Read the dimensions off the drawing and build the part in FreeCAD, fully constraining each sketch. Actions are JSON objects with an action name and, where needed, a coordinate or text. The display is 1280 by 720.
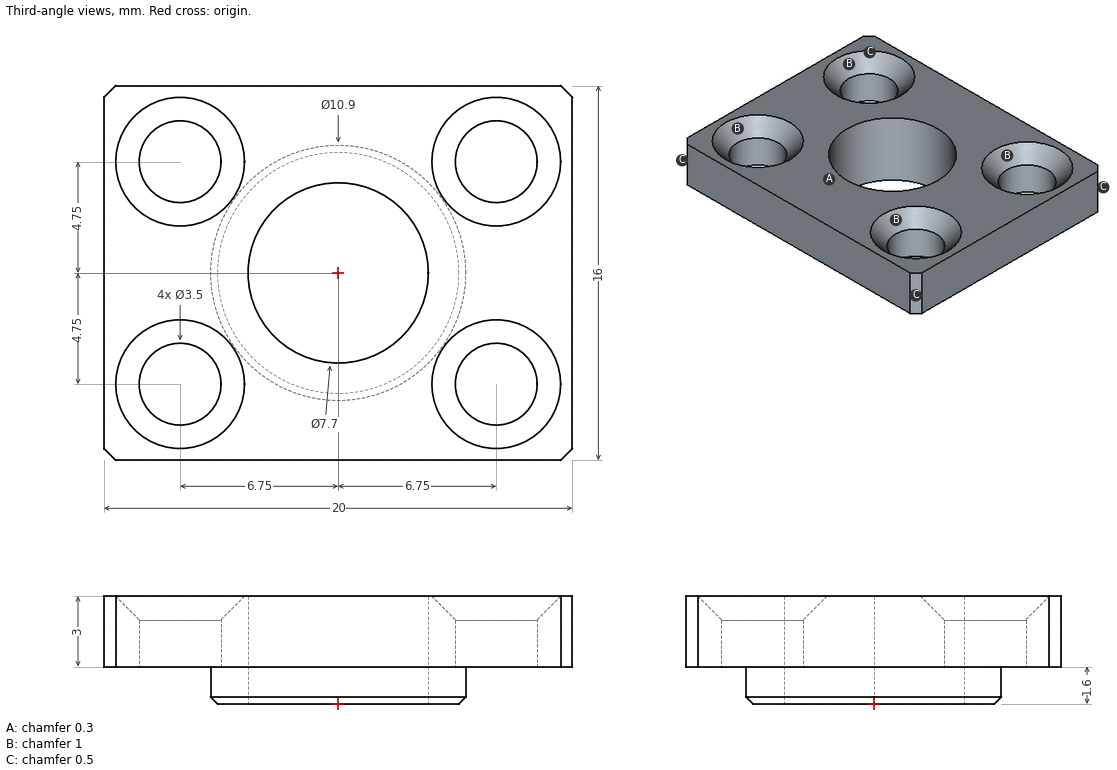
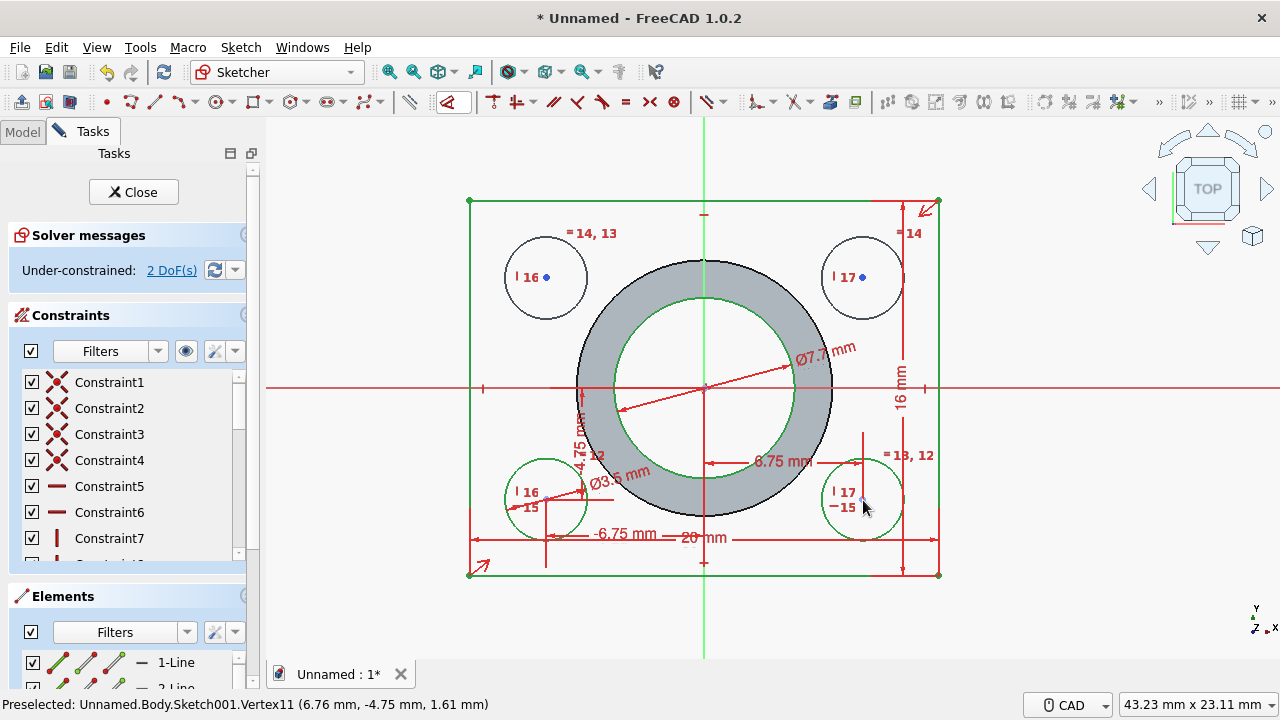
{"action": "left_click", "coordinate": [546, 278]}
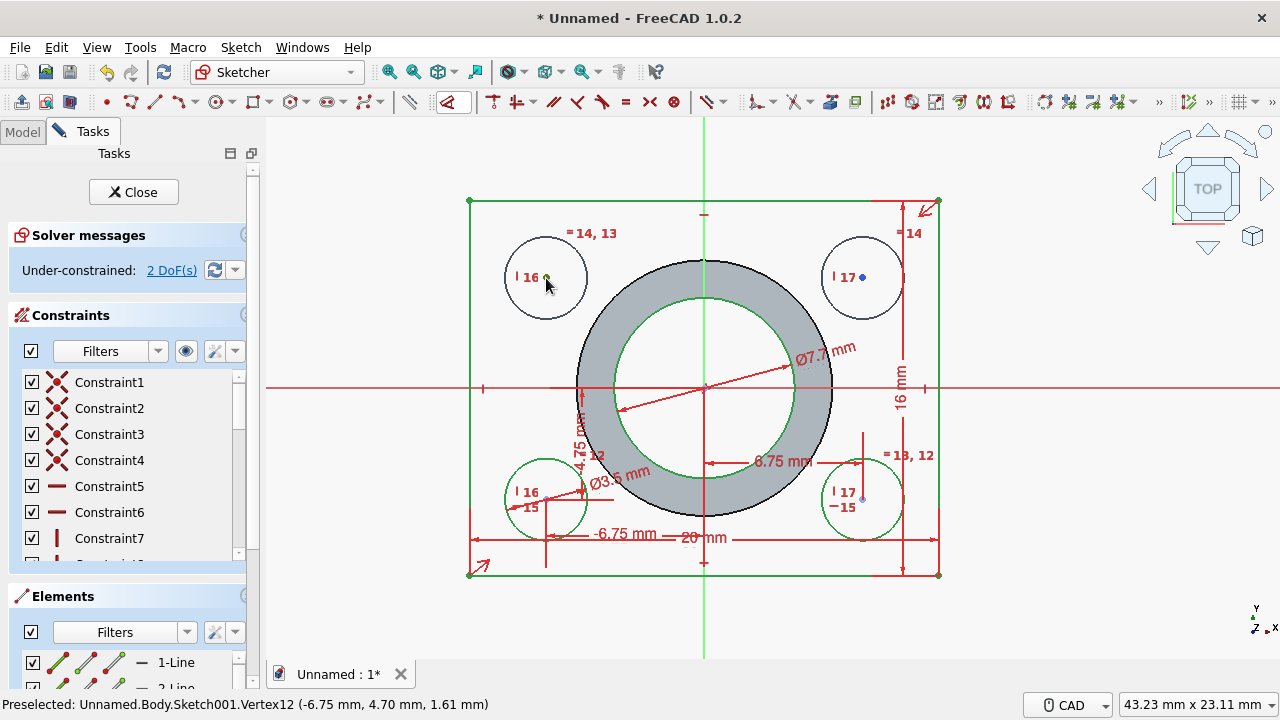
{"action": "key", "text": "i"}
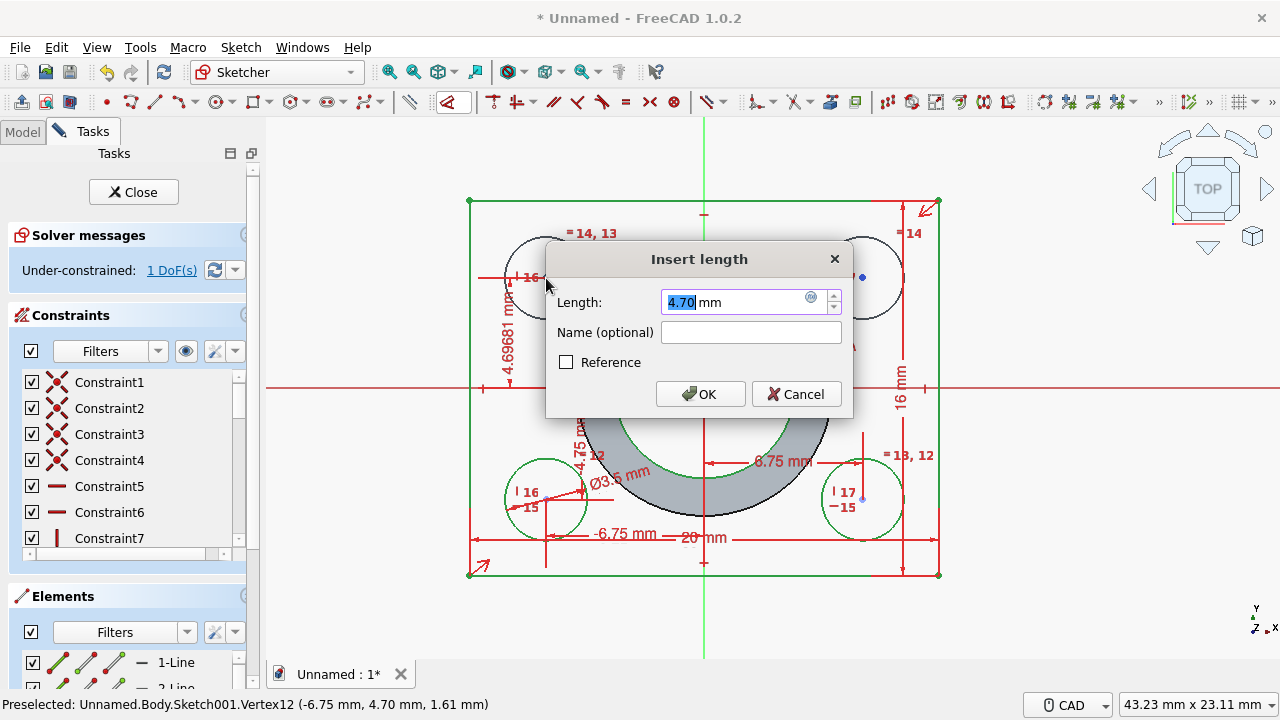
{"action": "type", "text": "4.75"}
{"action": "key", "text": "Return"}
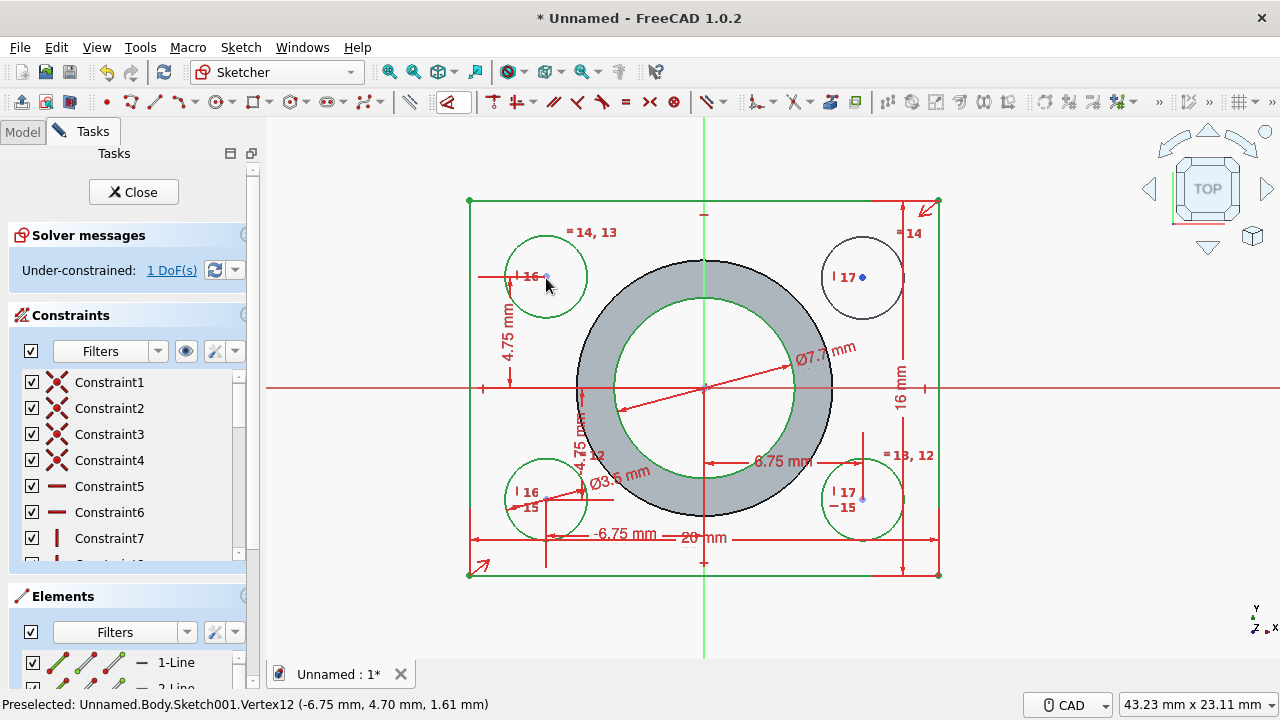
{"action": "left_click", "coordinate": [863, 278]}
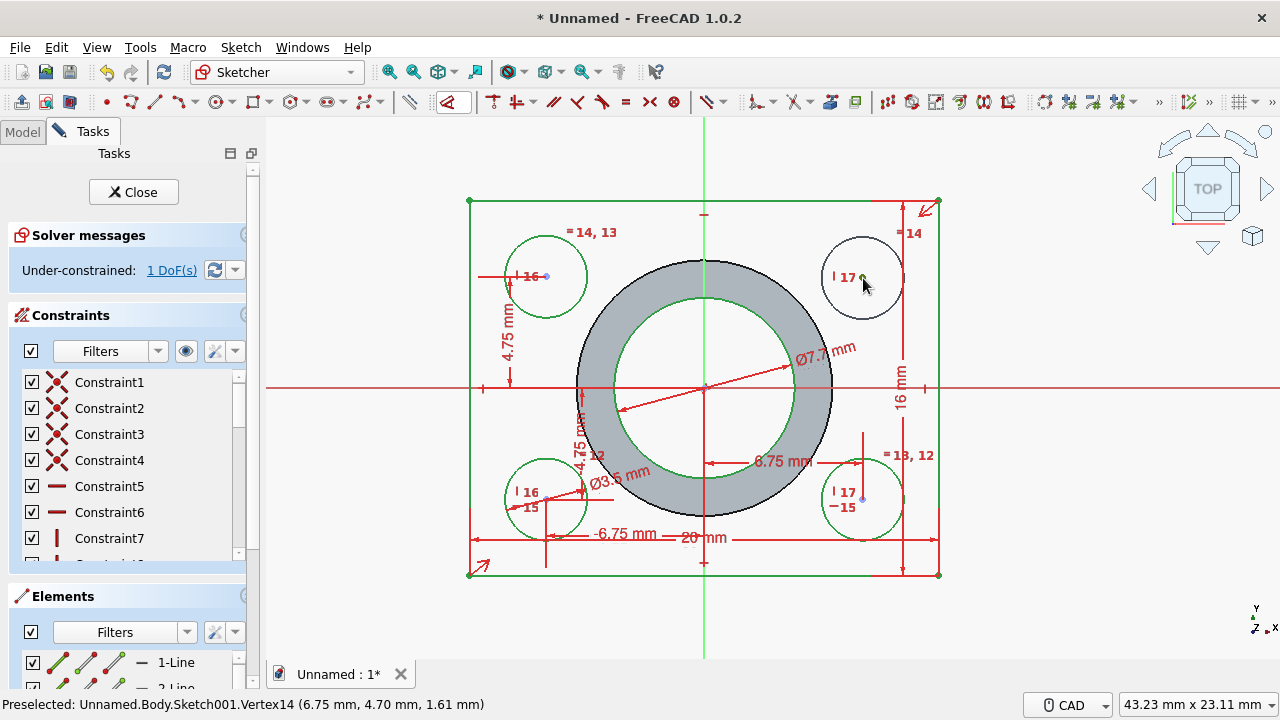
{"action": "key", "text": "i"}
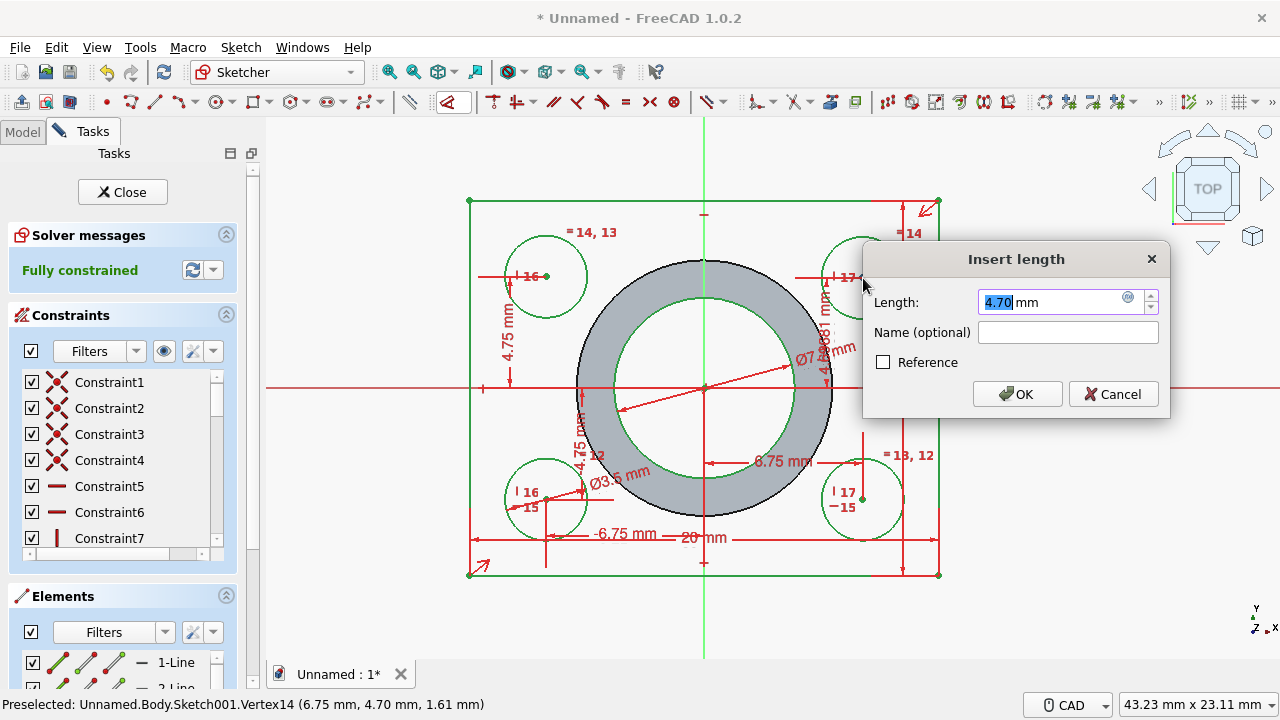
{"action": "type", "text": "4.75"}
{"action": "key", "text": "Return"}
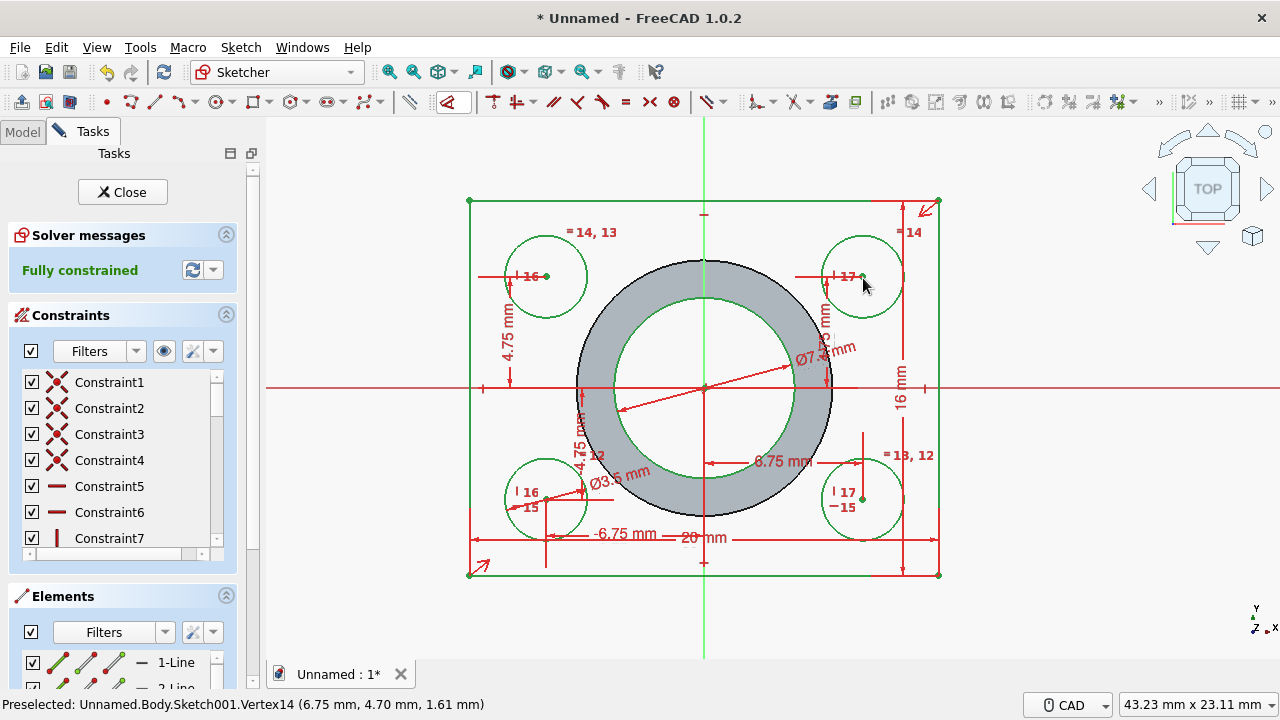
{"action": "left_click", "coordinate": [123, 192]}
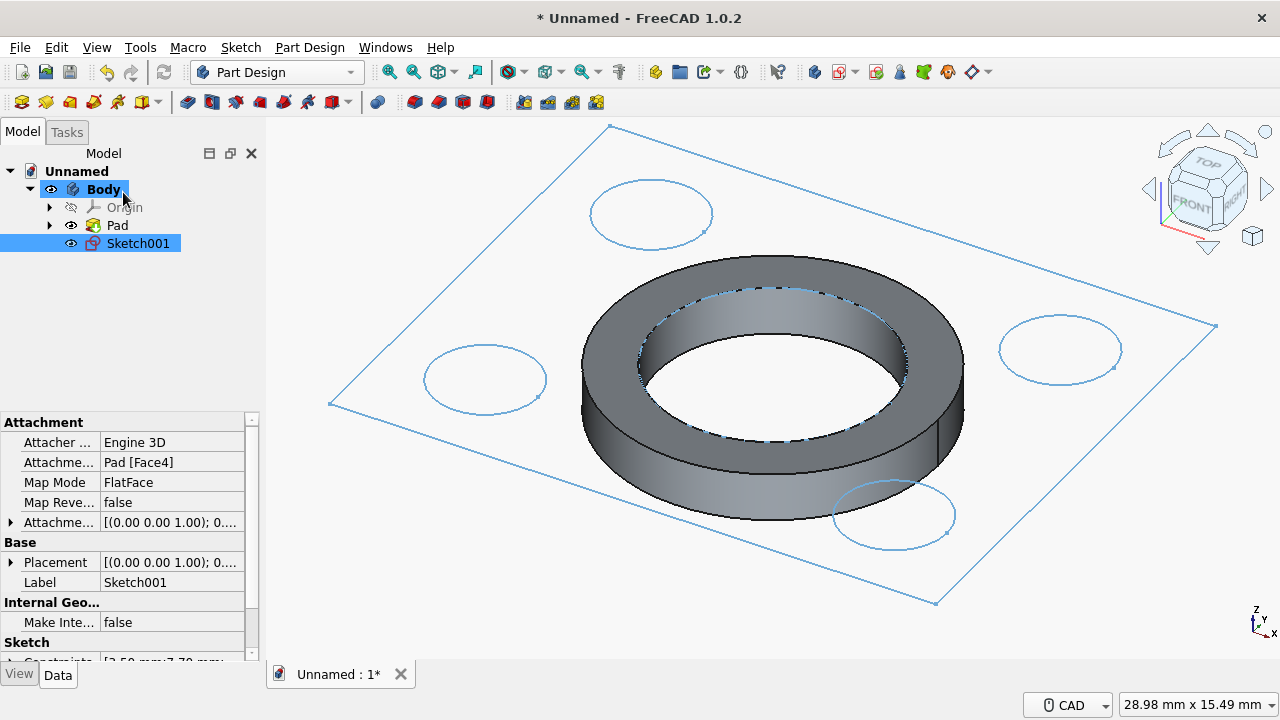
{"action": "left_click", "coordinate": [22, 102]}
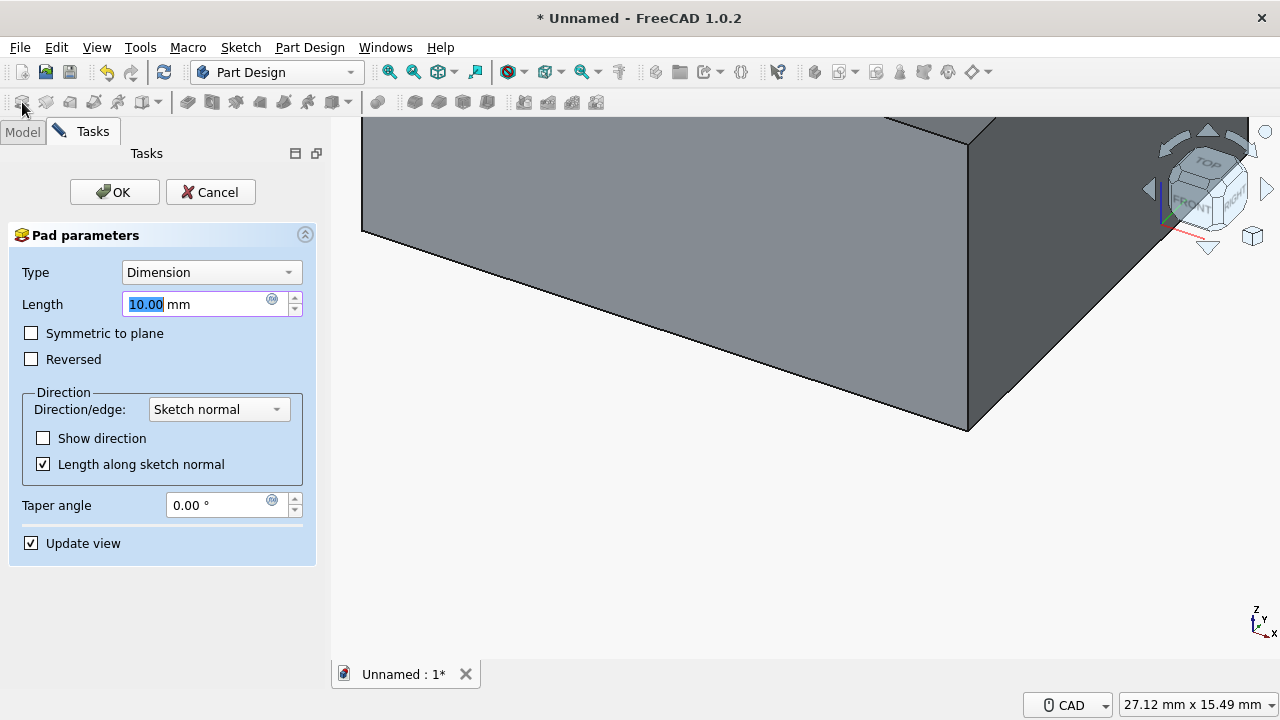
{"action": "type", "text": "3"}
{"action": "key", "text": "Tab"}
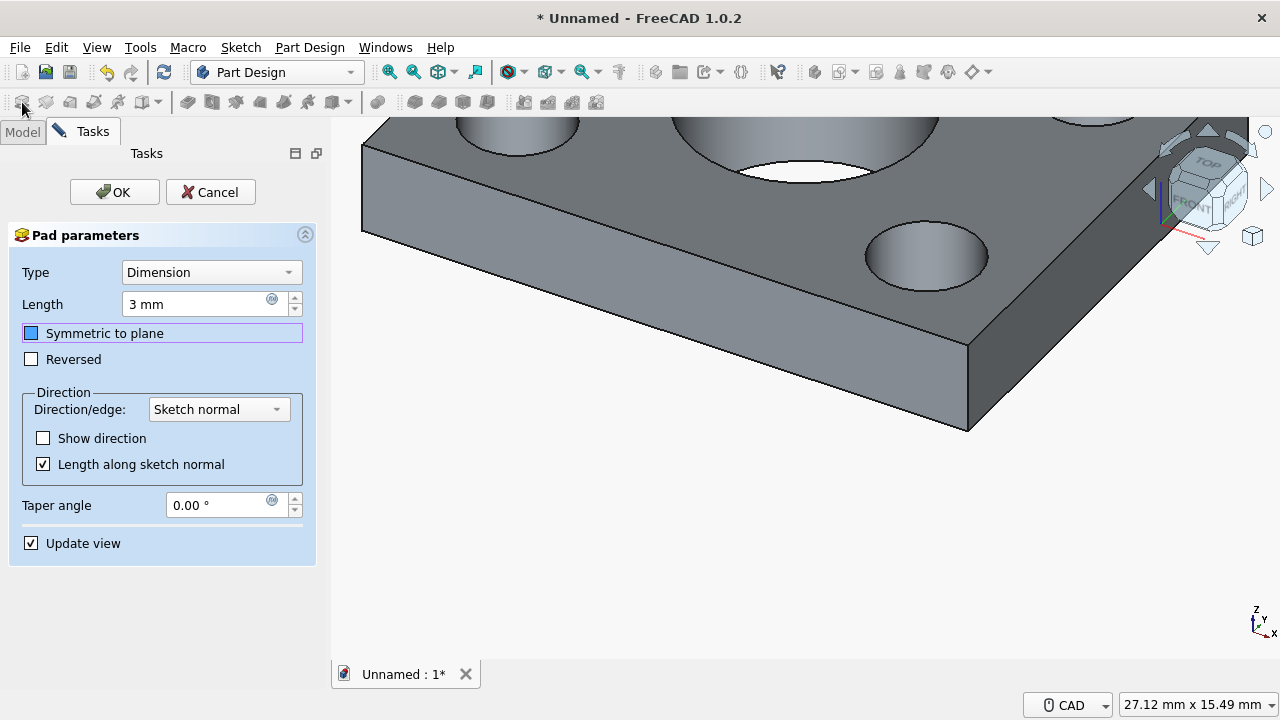
{"action": "left_click", "coordinate": [115, 192]}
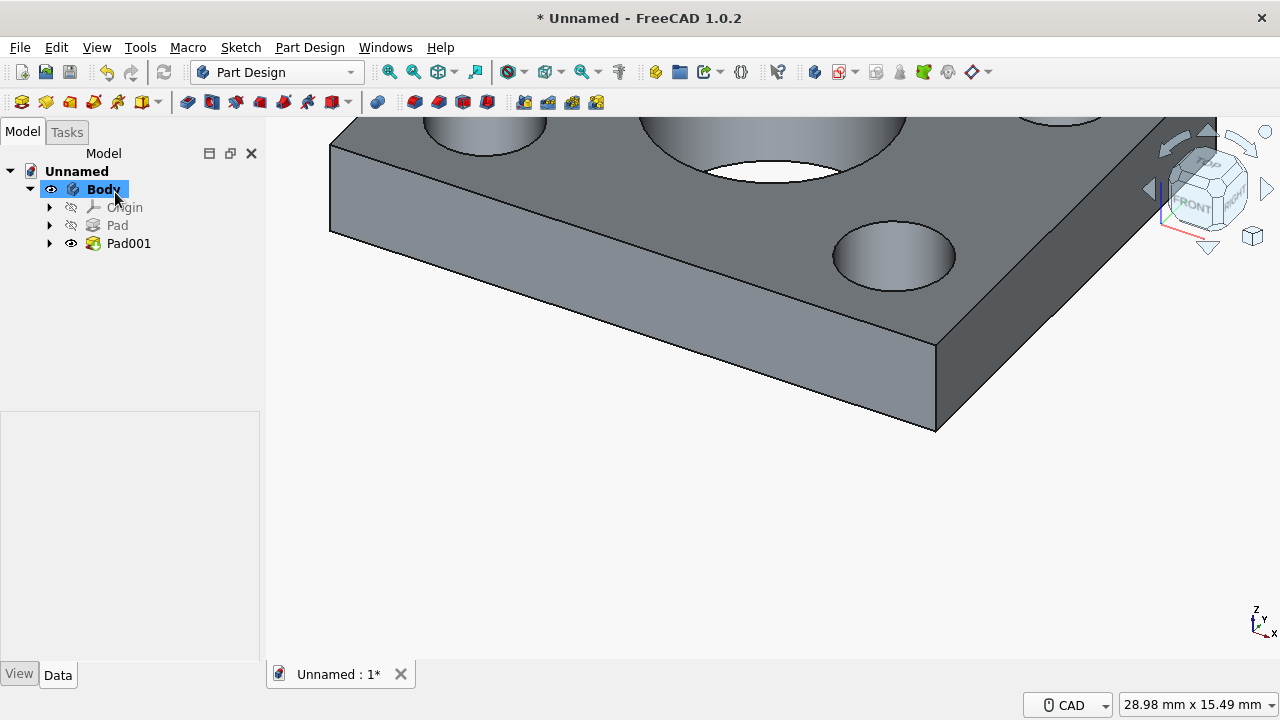
{"action": "left_click", "coordinate": [390, 72]}